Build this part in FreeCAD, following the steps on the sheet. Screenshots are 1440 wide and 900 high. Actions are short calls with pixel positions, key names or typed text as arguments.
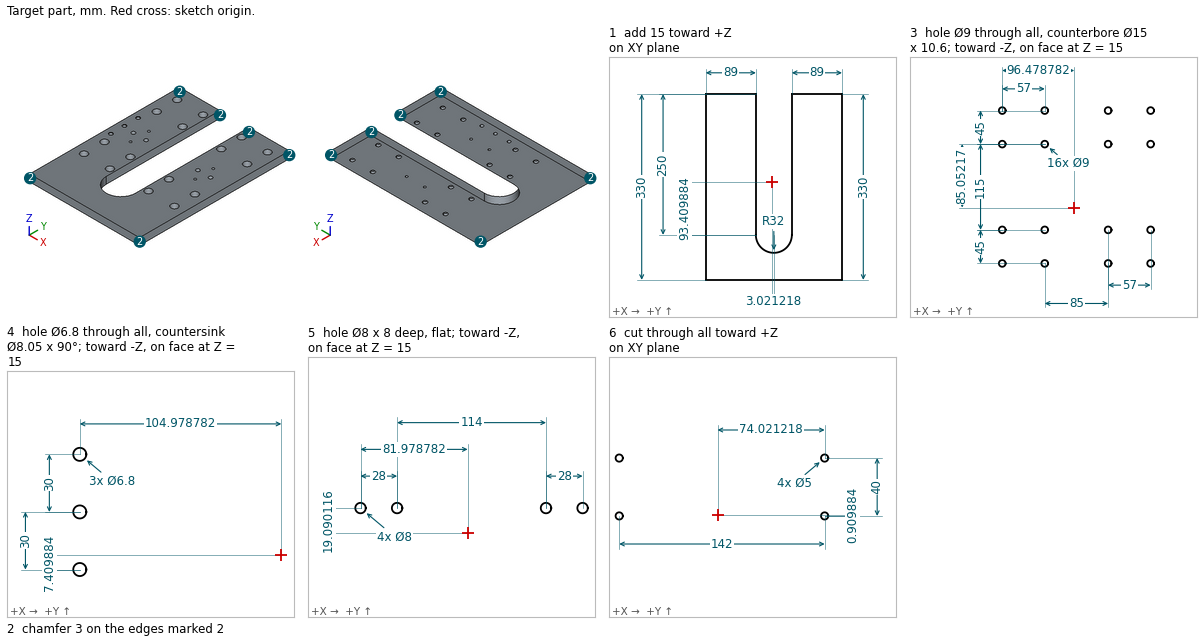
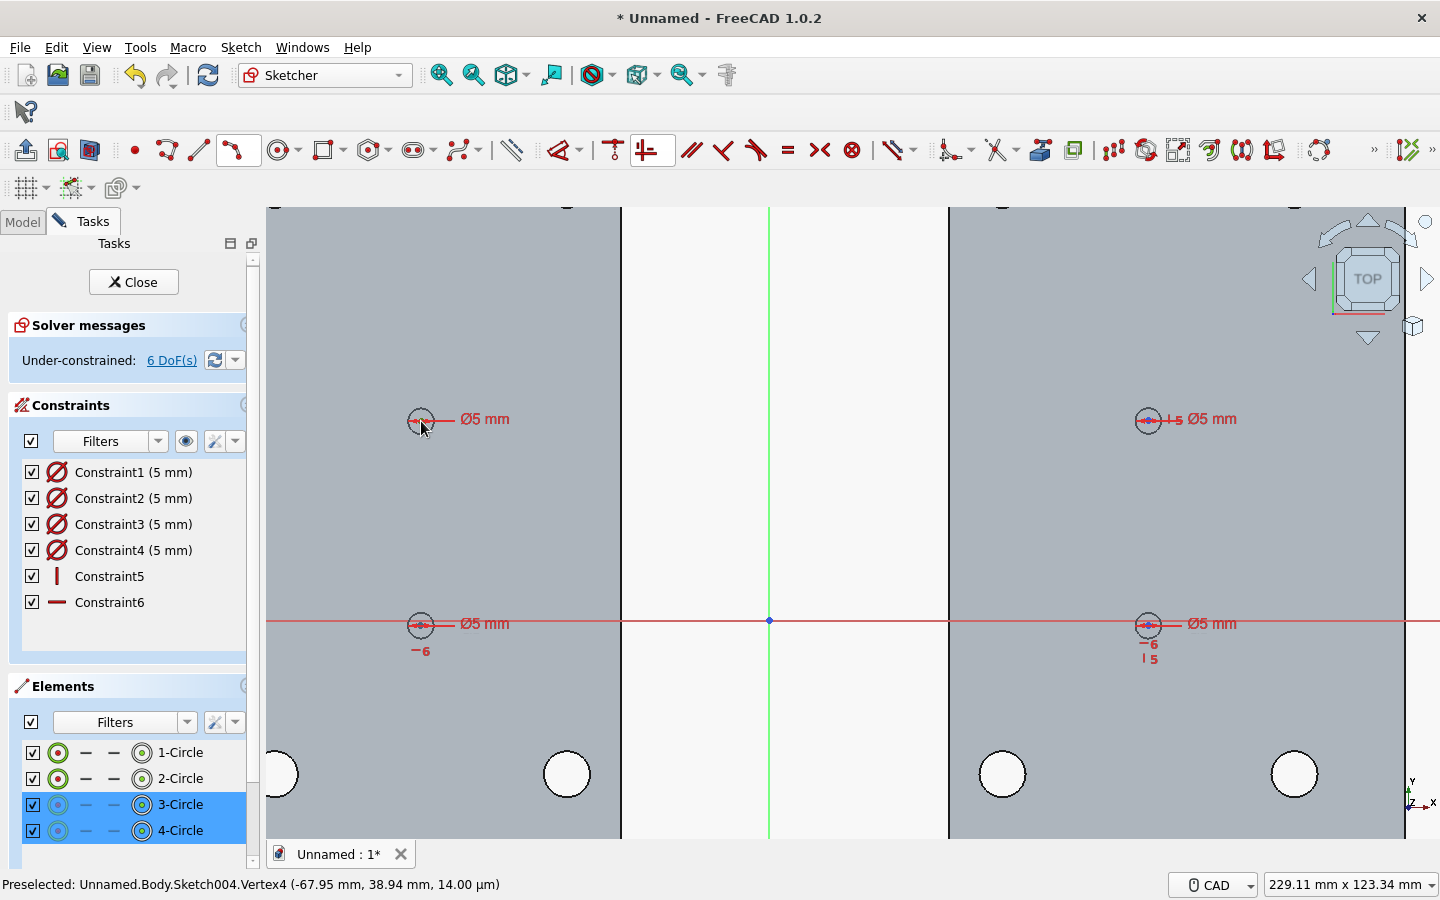
key(v)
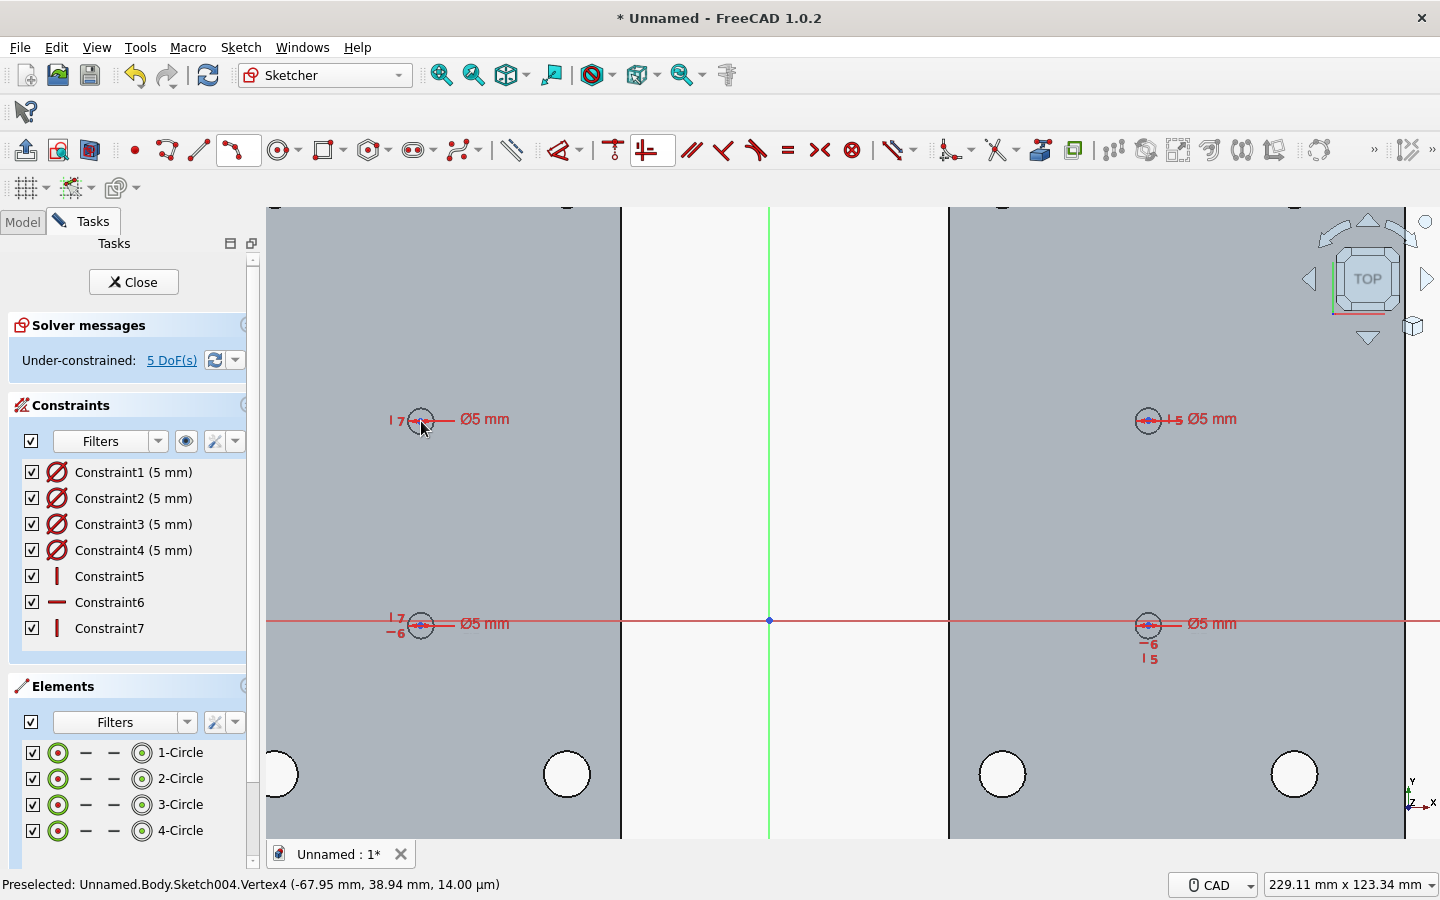
click(1148, 421)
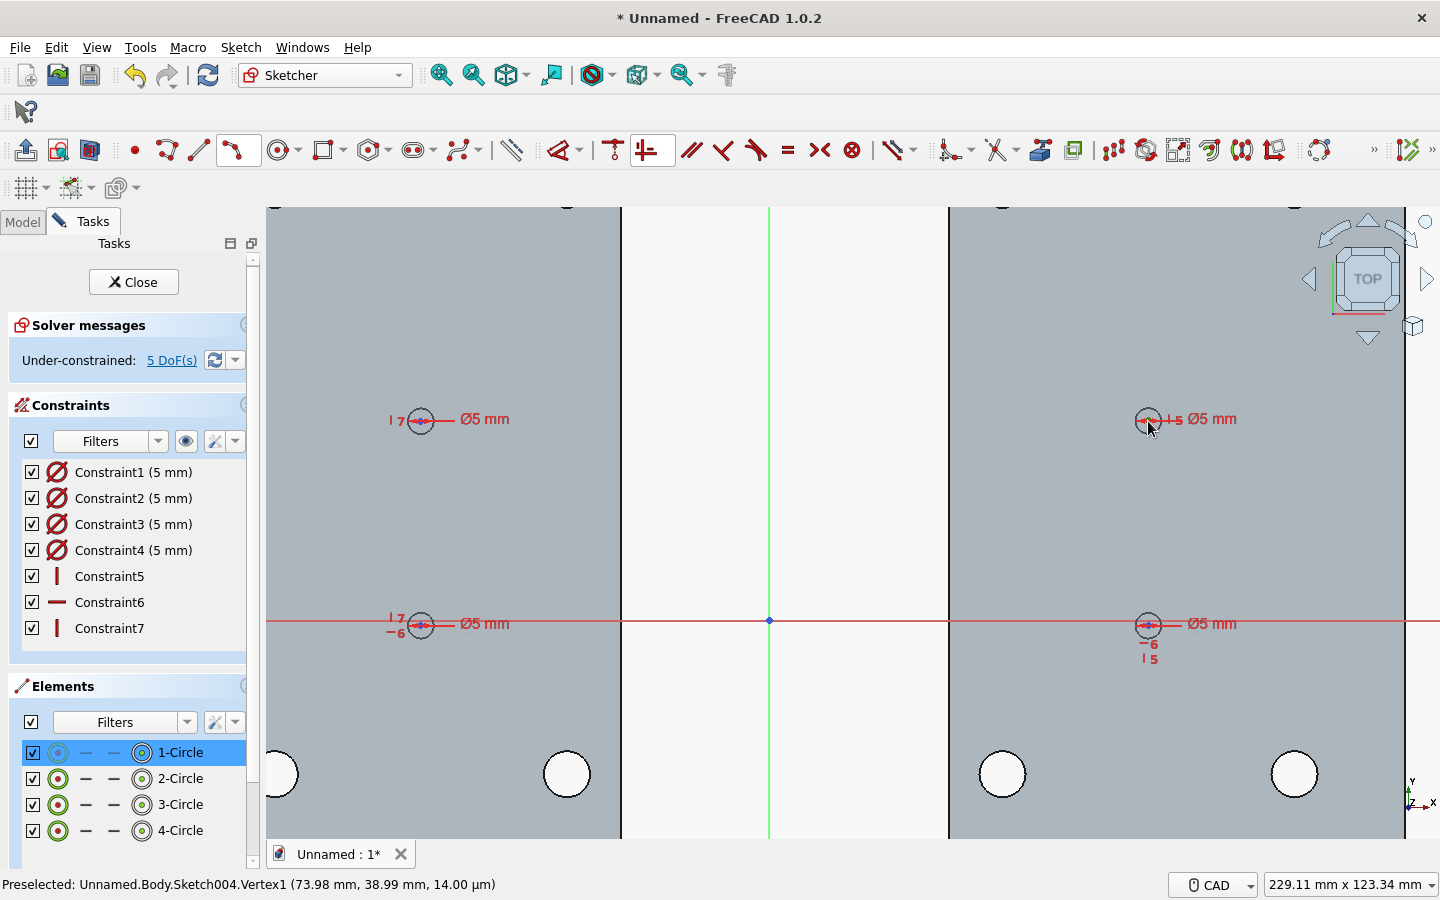
click(421, 421)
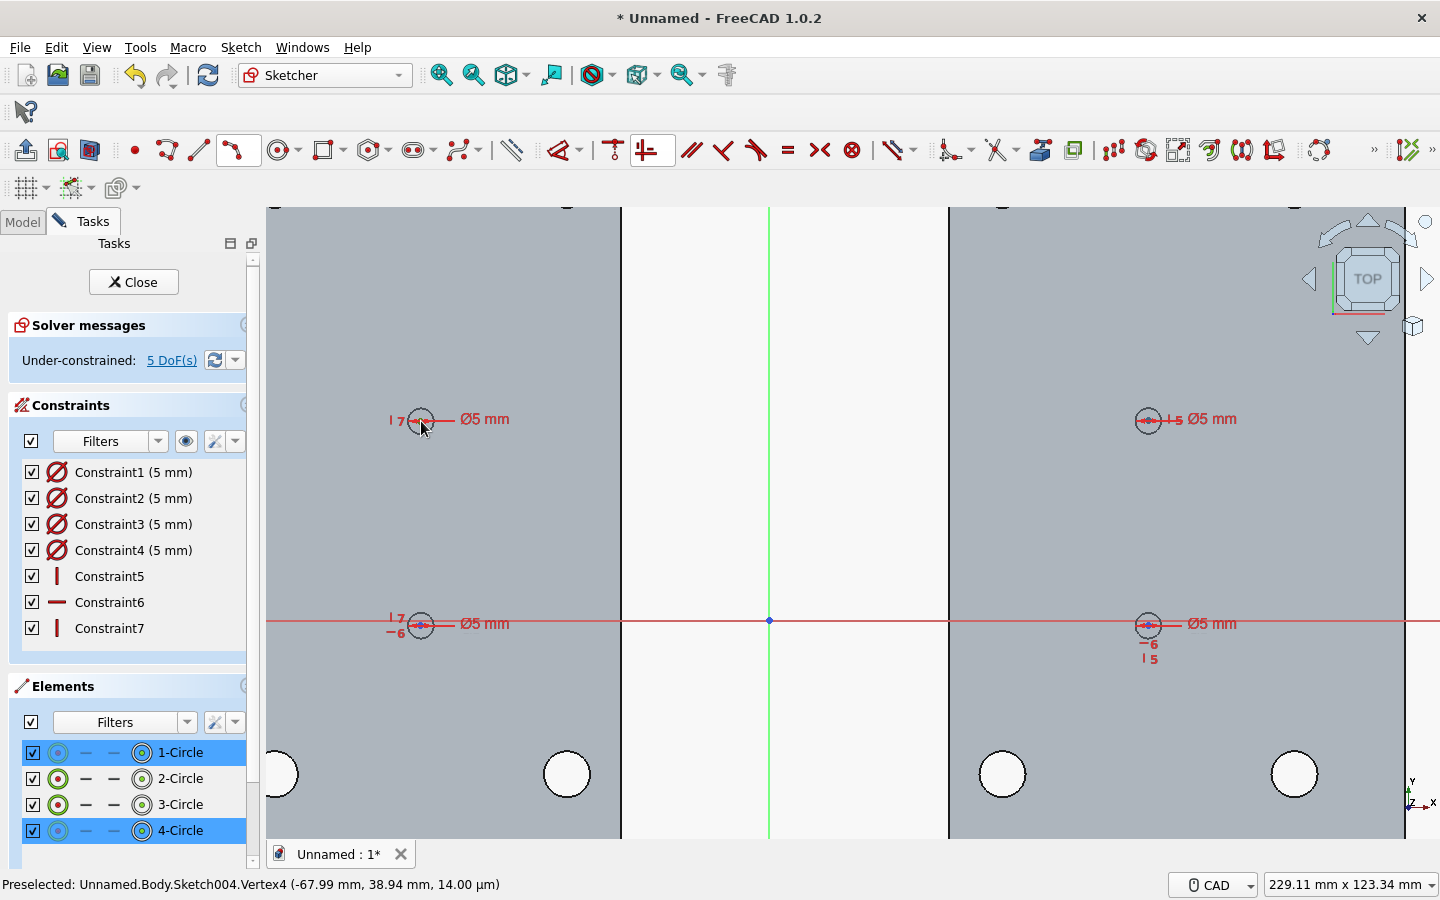
click(670, 150)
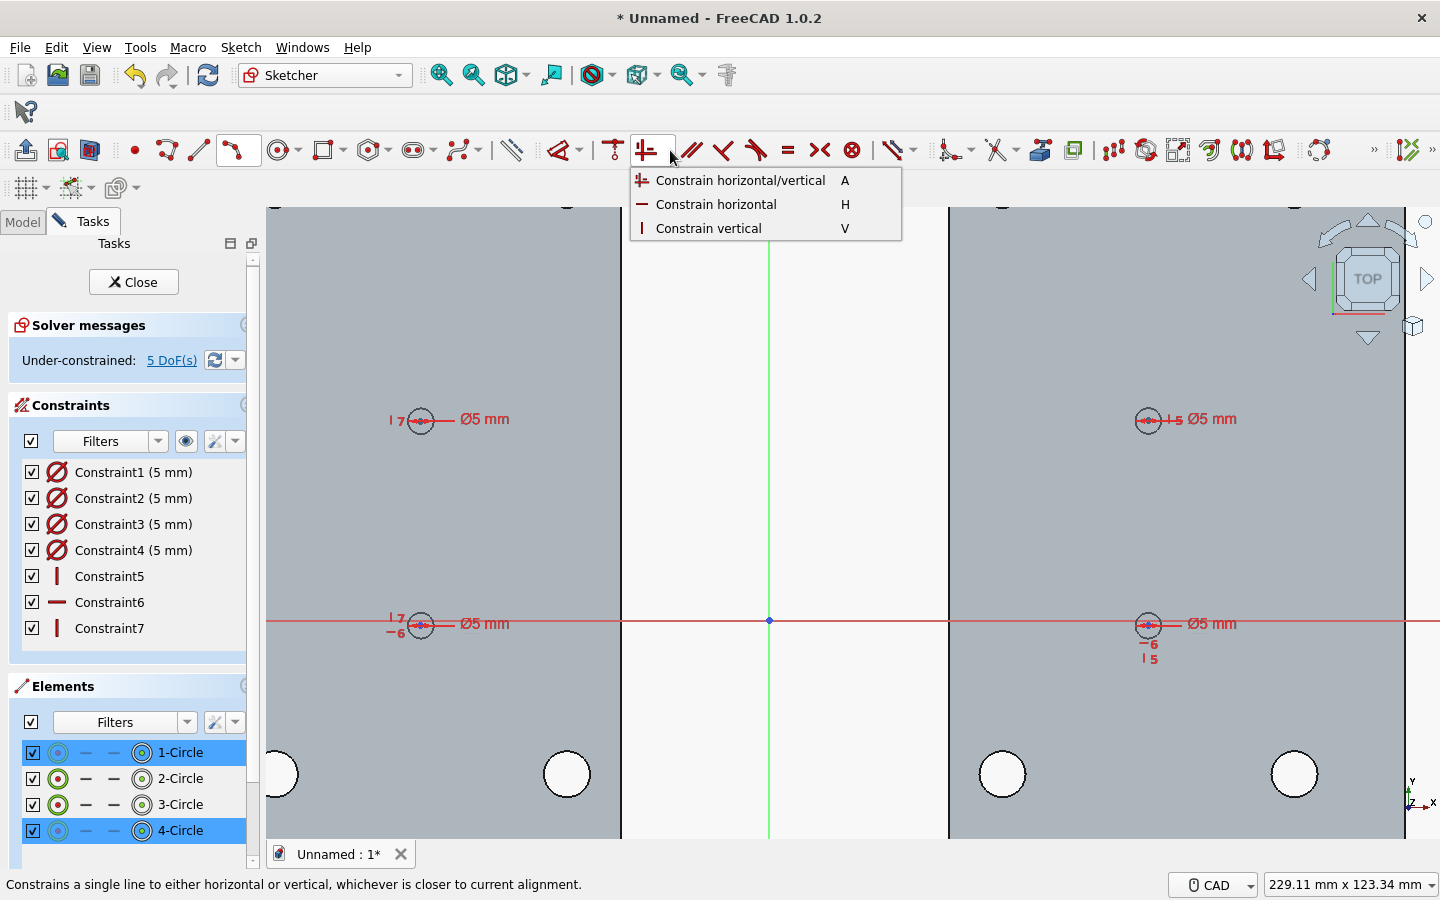
click(766, 204)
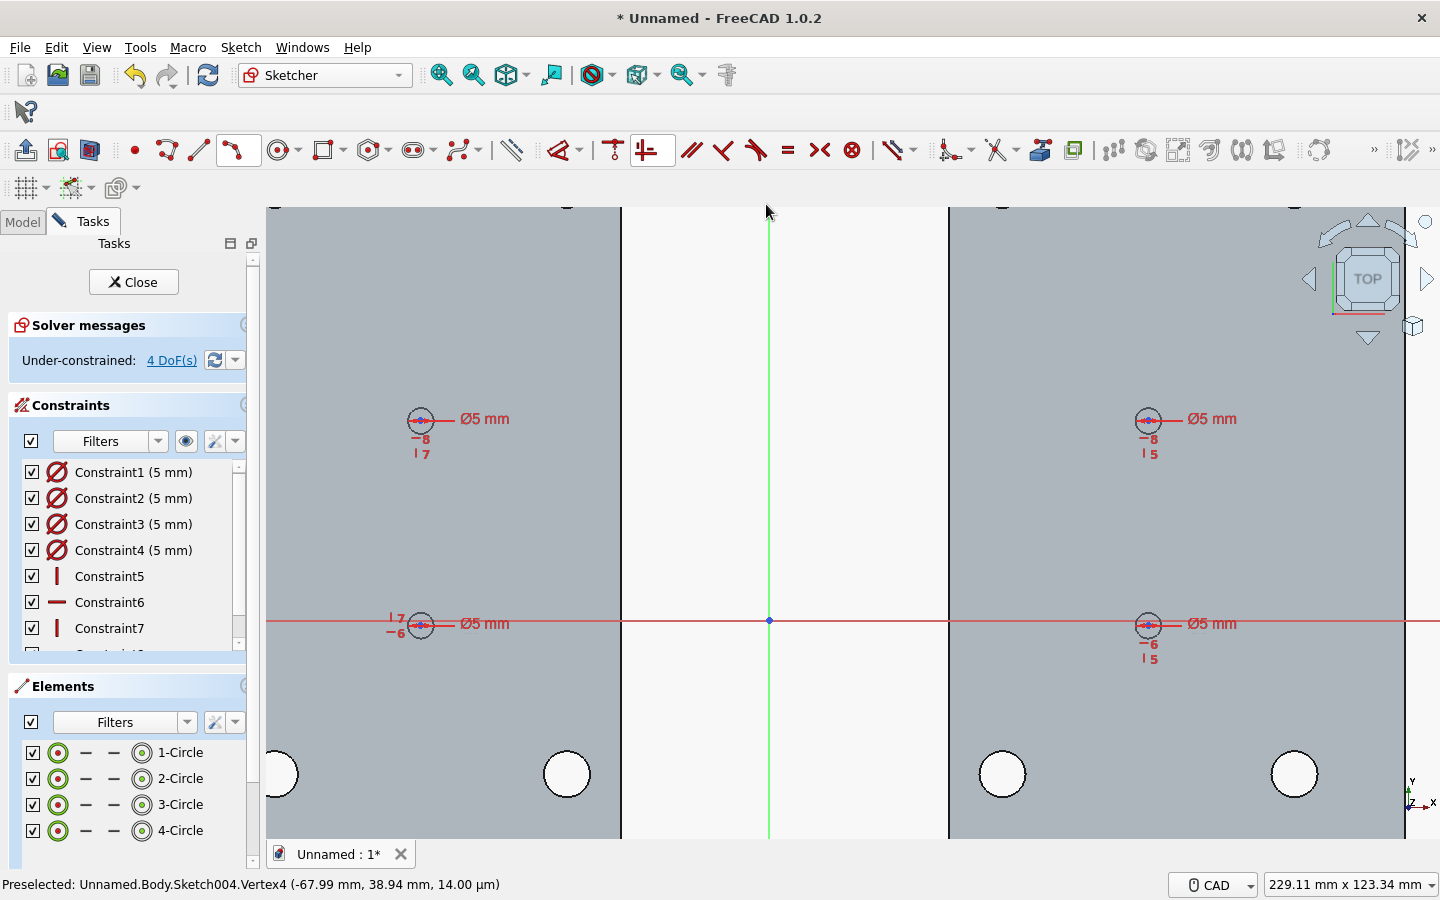
key(d)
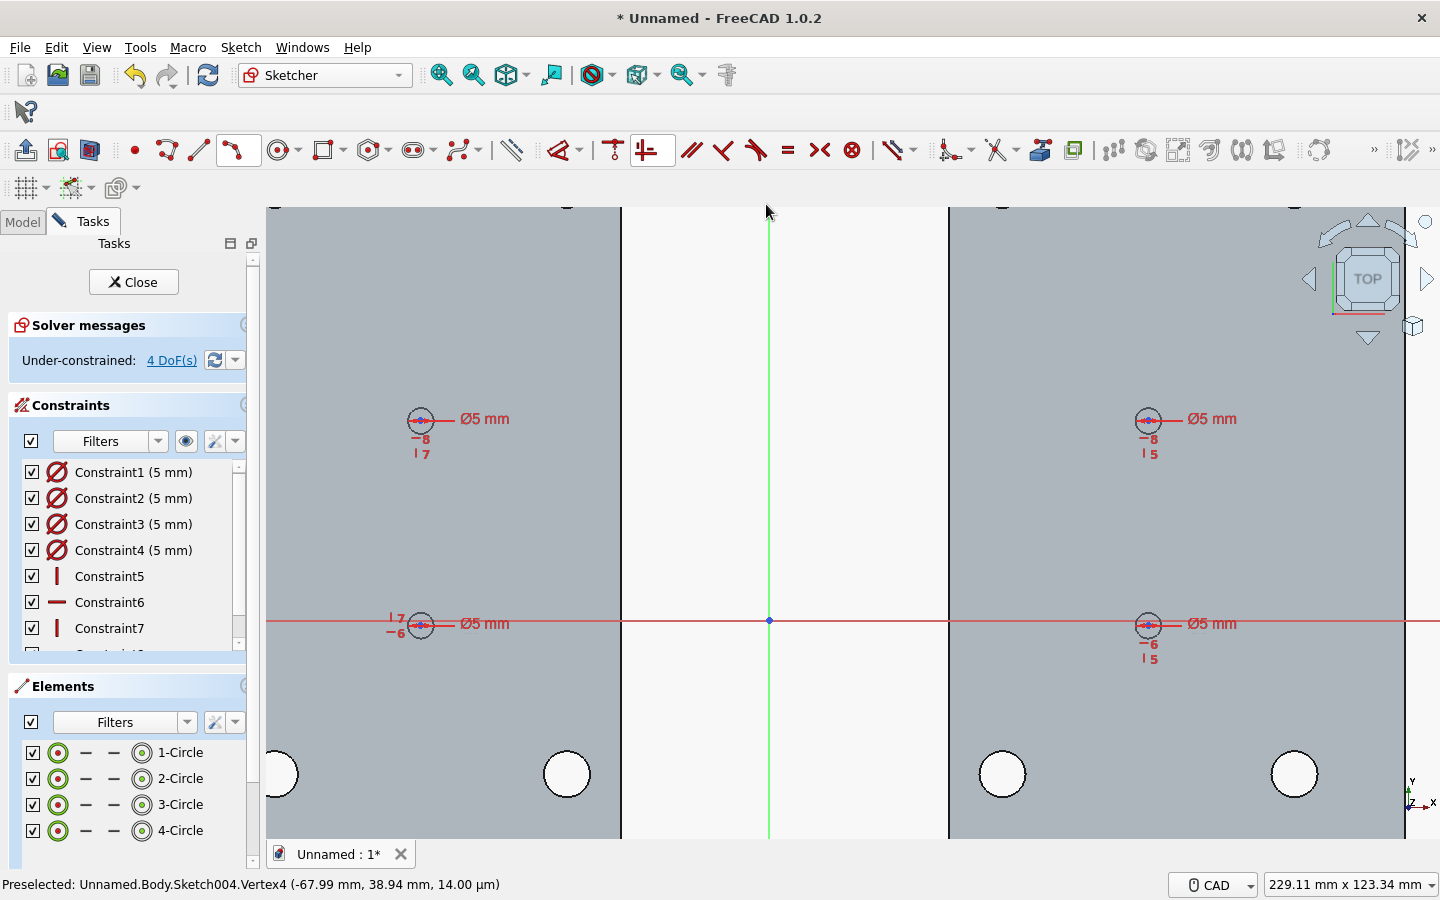
click(1148, 421)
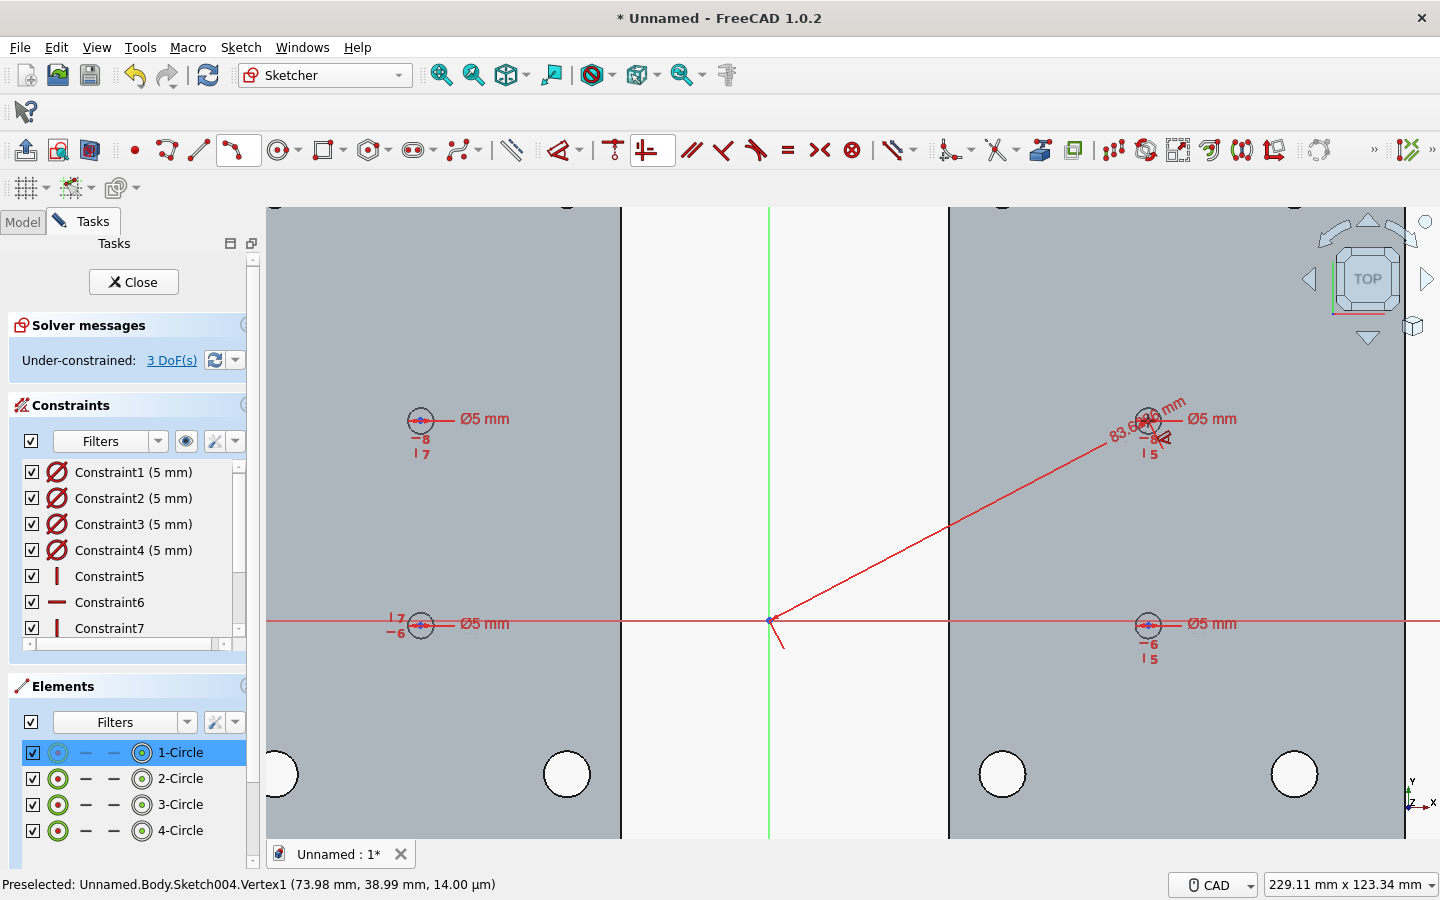
click(1148, 626)
click(1182, 523)